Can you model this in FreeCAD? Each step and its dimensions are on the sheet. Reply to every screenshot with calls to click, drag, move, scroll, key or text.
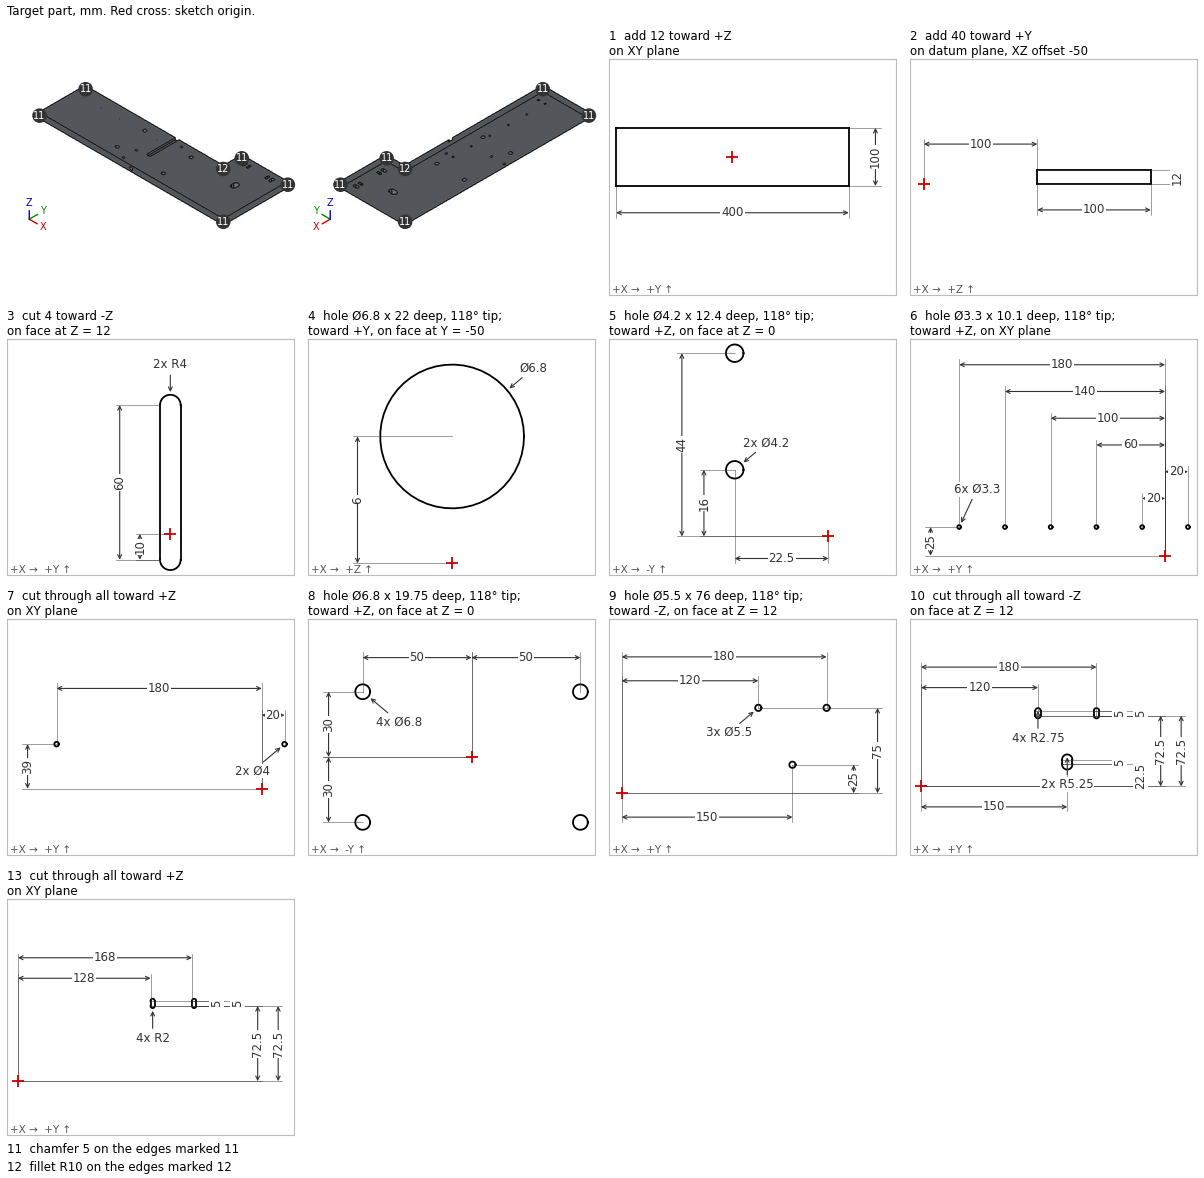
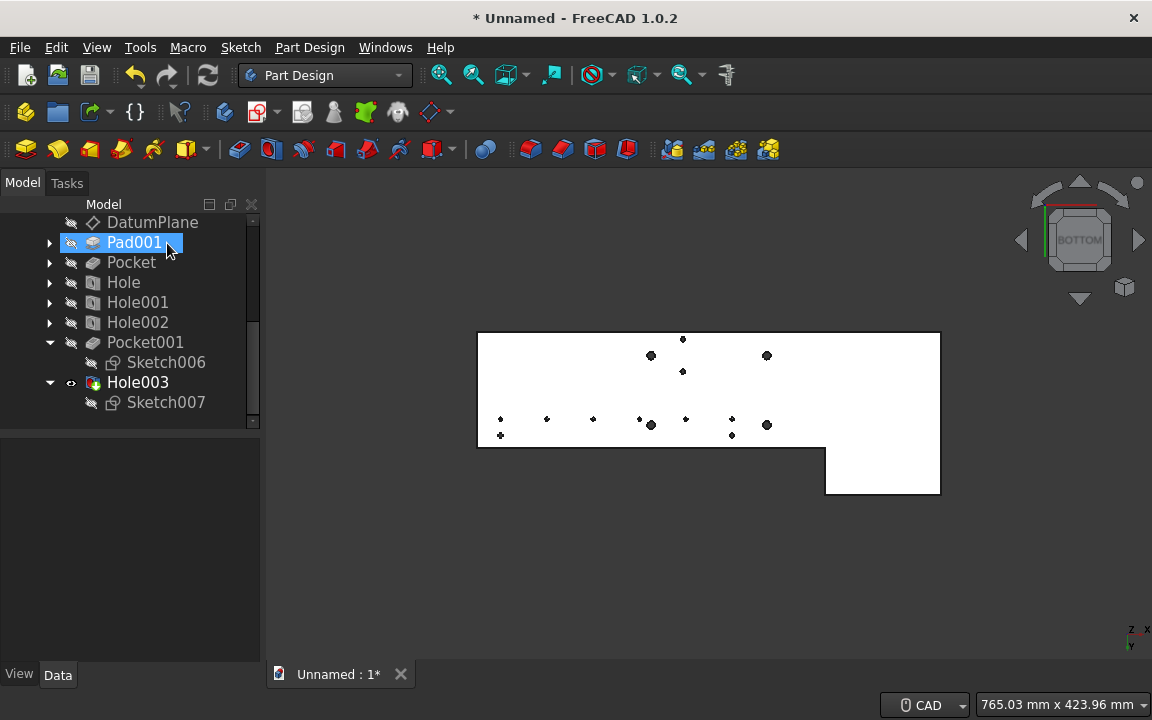
key(0)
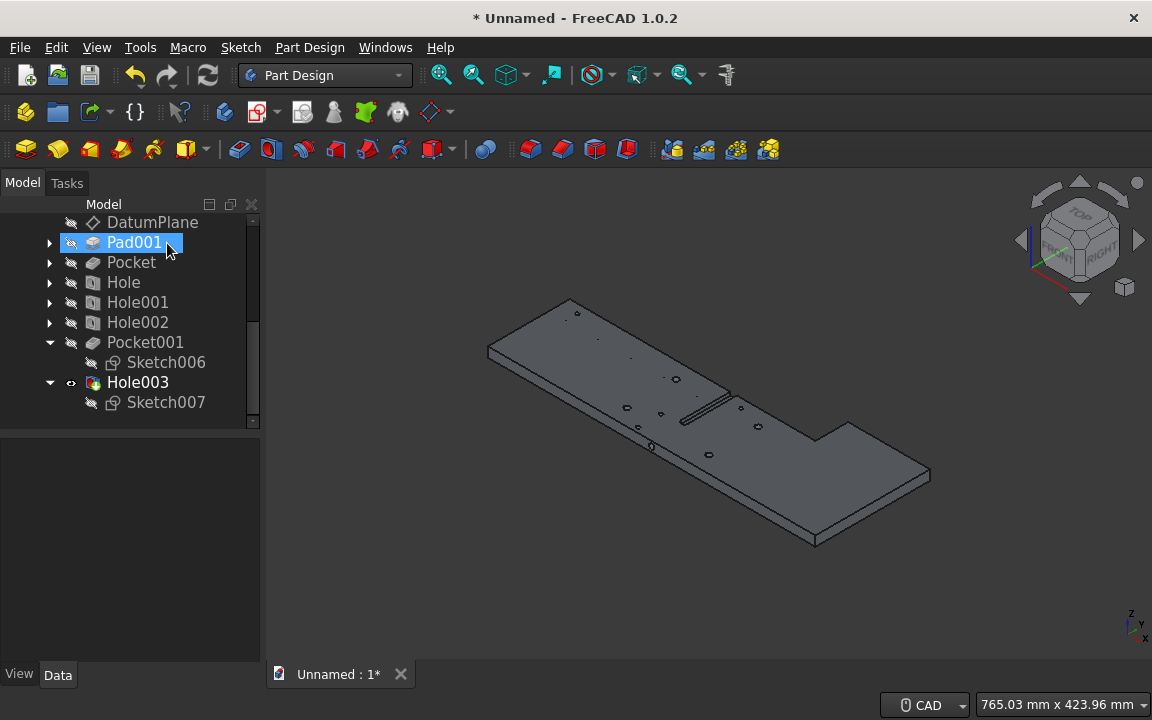
click(786, 470)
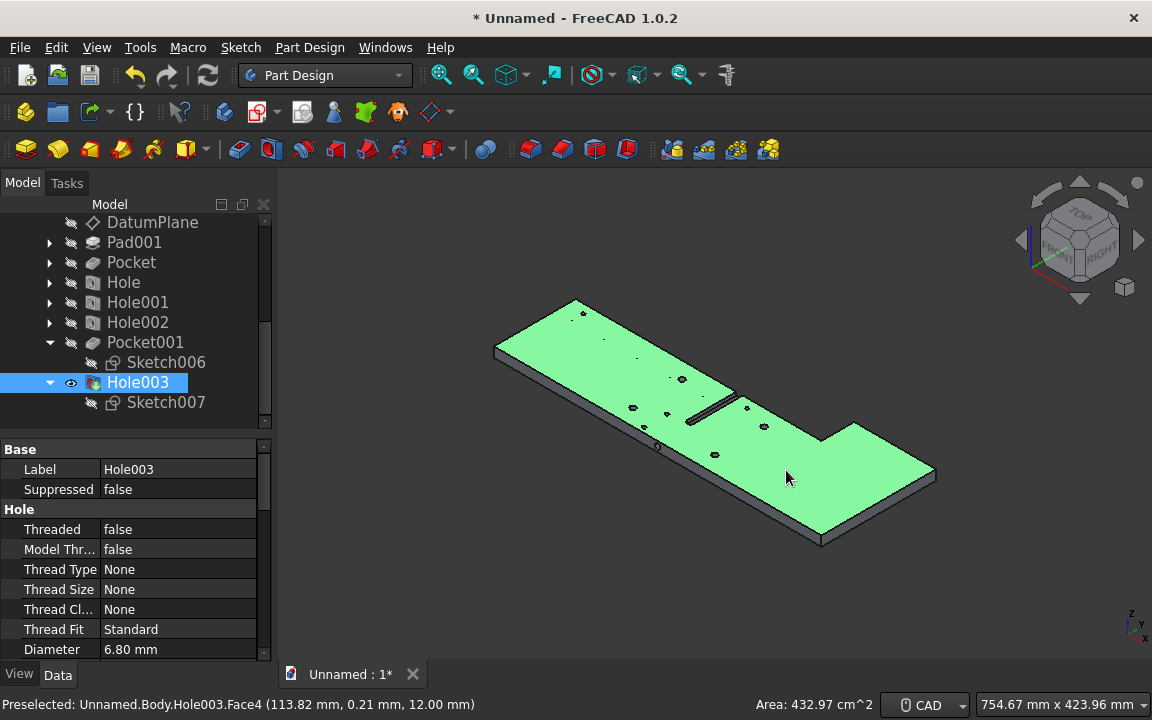
click(258, 112)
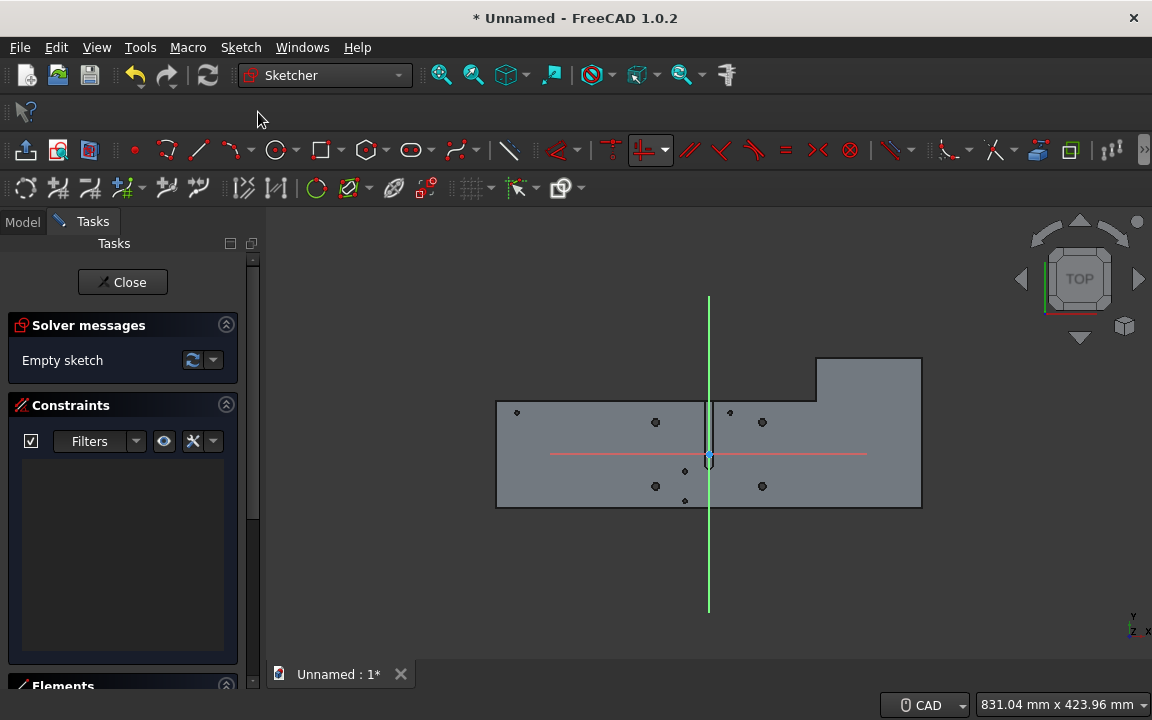
scroll(927, 393, up, 8)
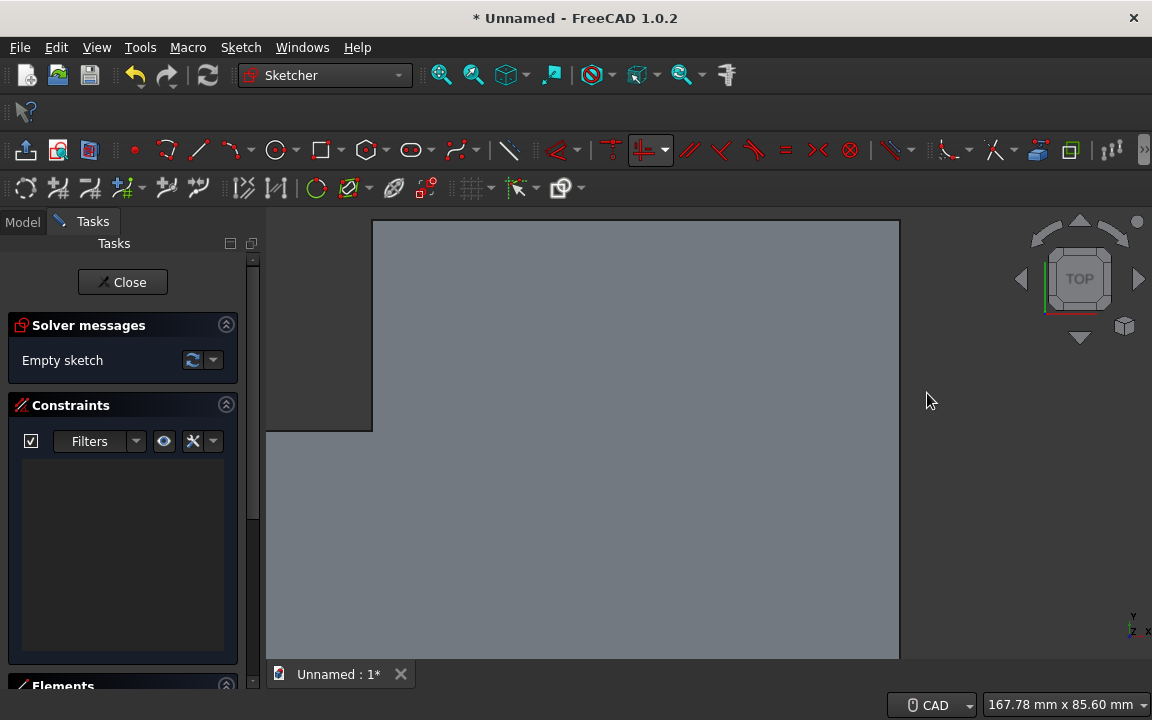
click(276, 150)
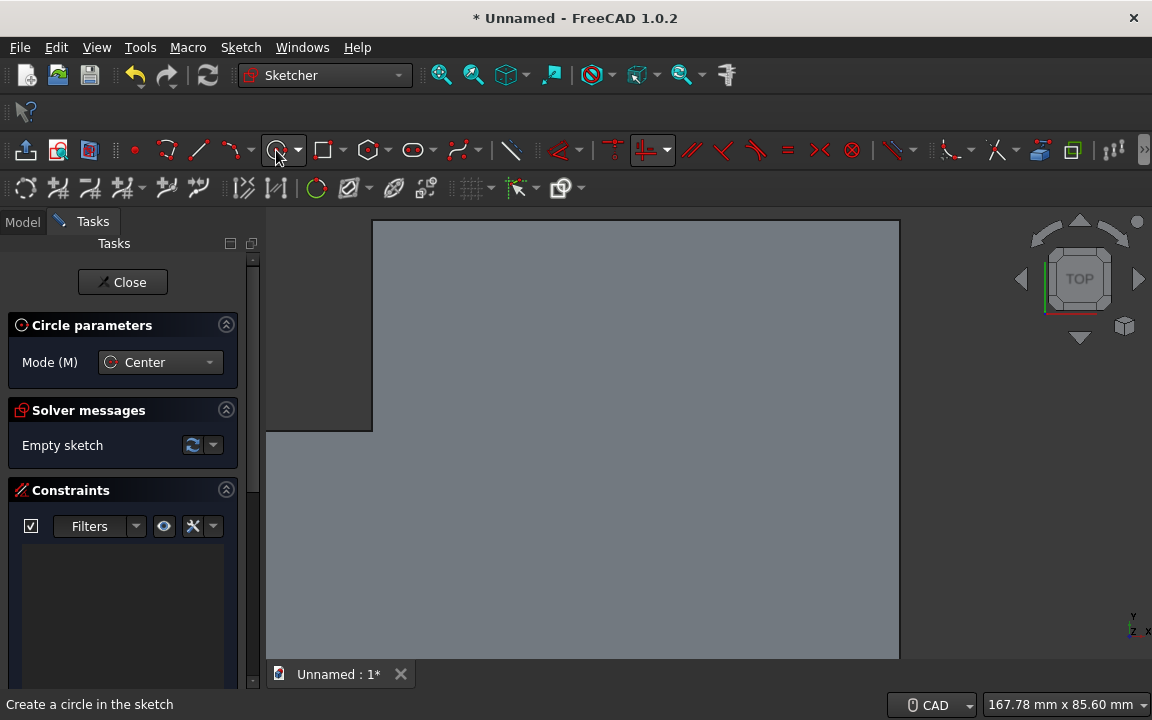
scroll(478, 299, up, 3)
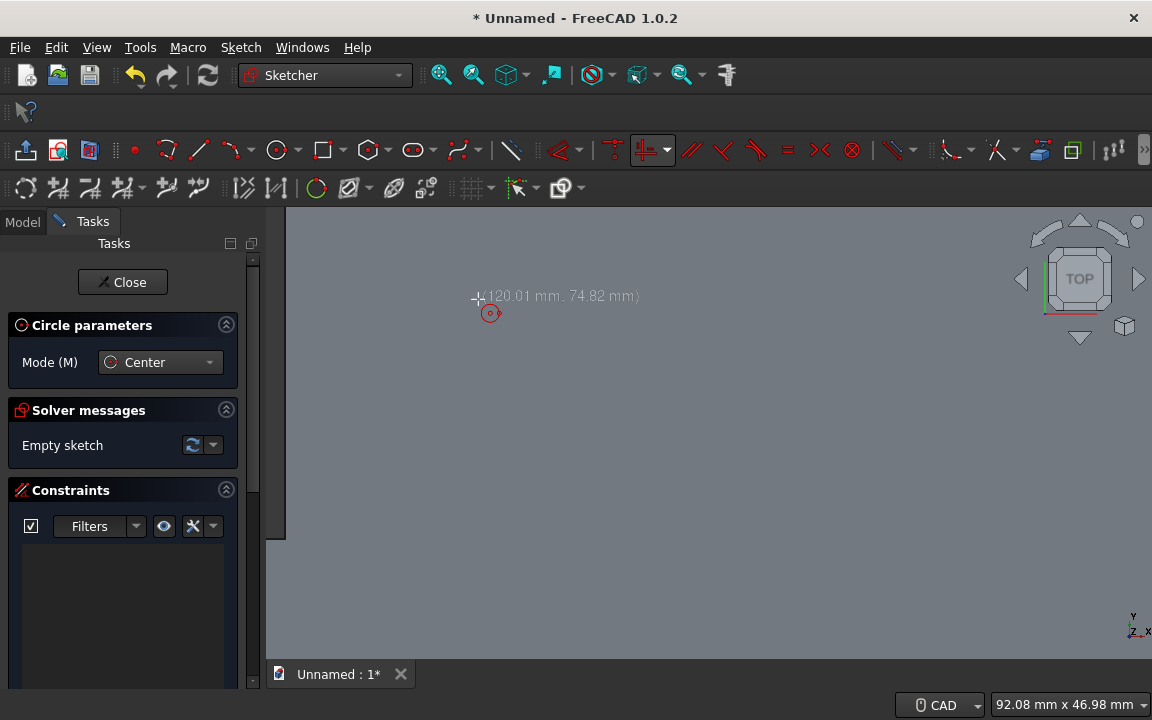
click(478, 299)
move(496, 280)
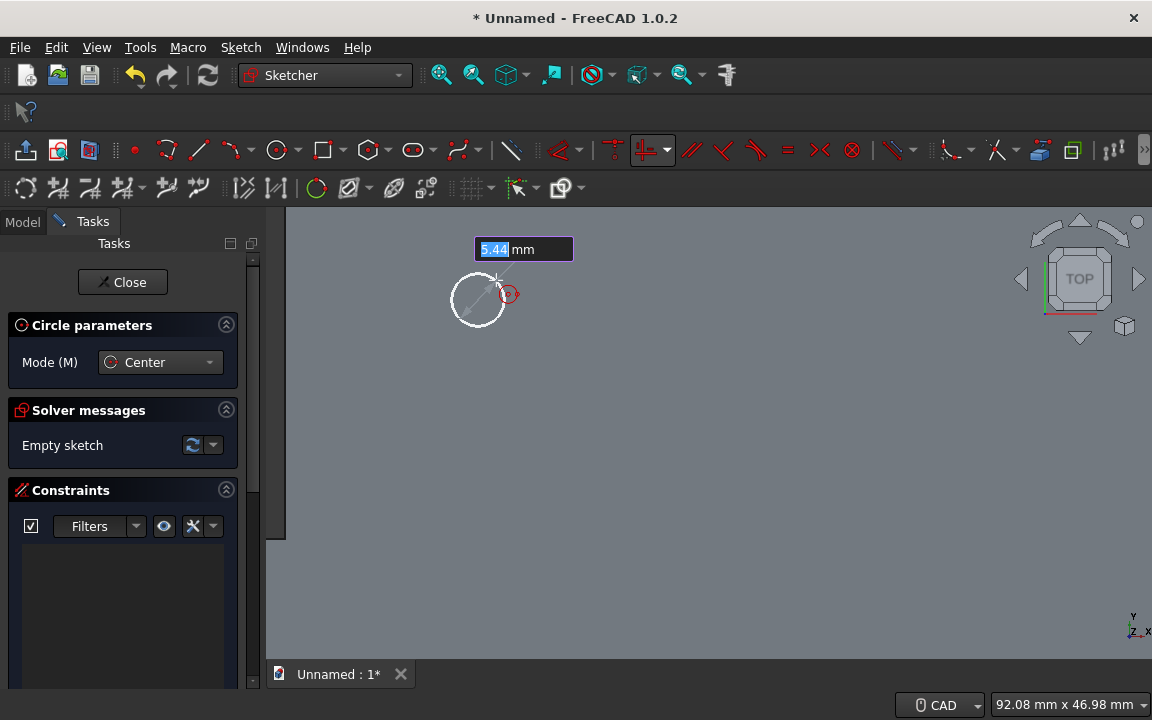
text(5.5)
key(Return)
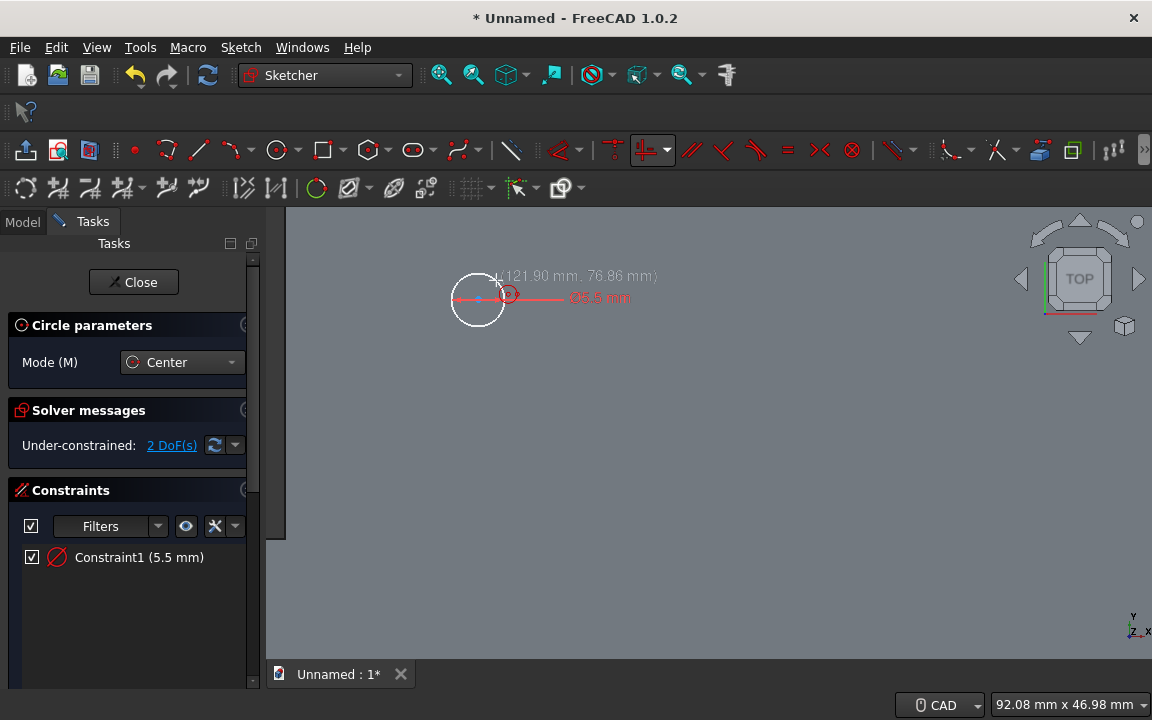
scroll(487, 303, down, 3)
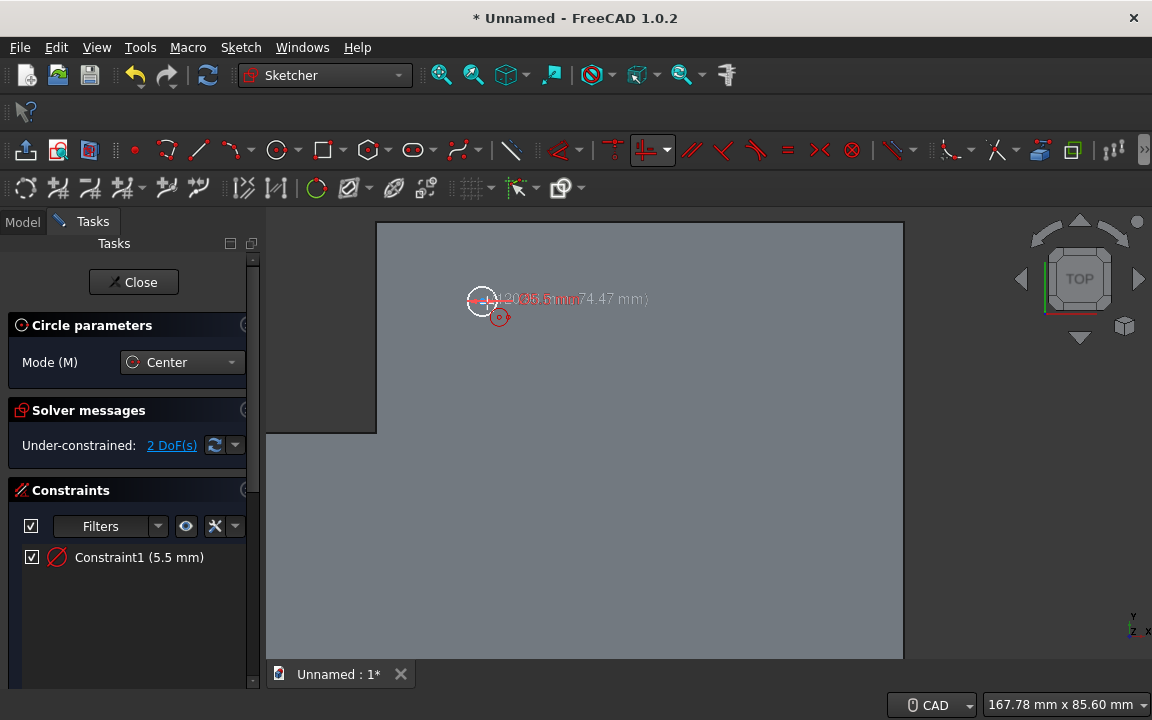
scroll(799, 301, up, 3)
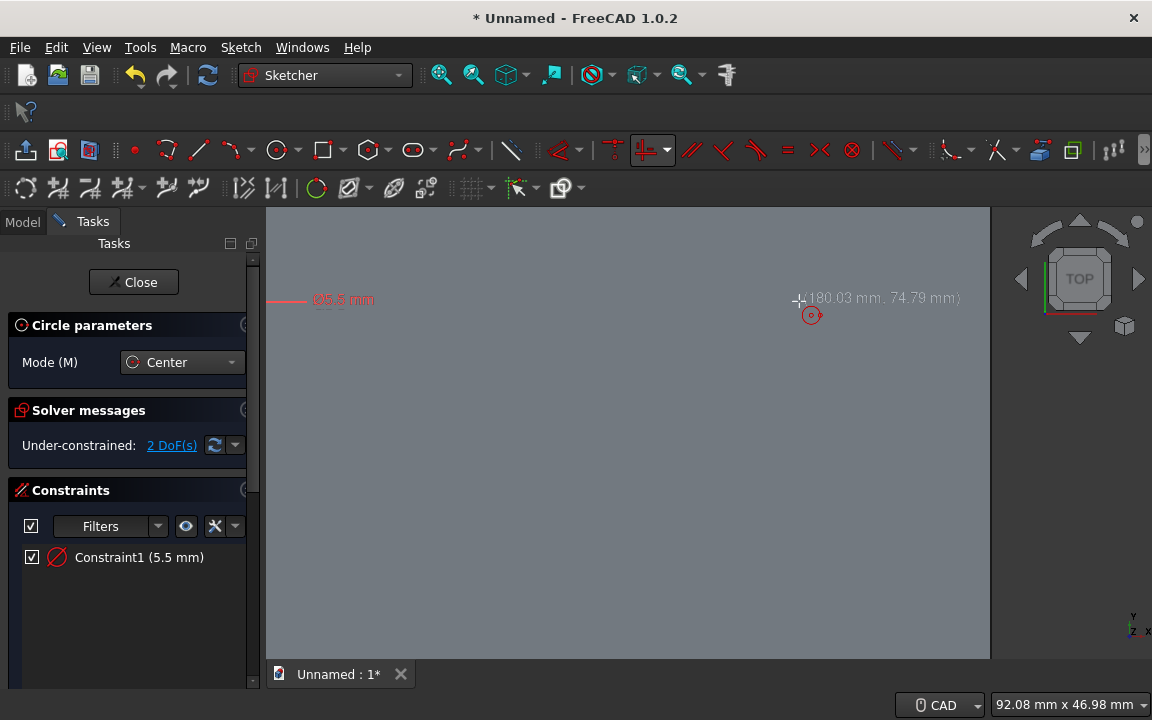
click(798, 301)
move(817, 282)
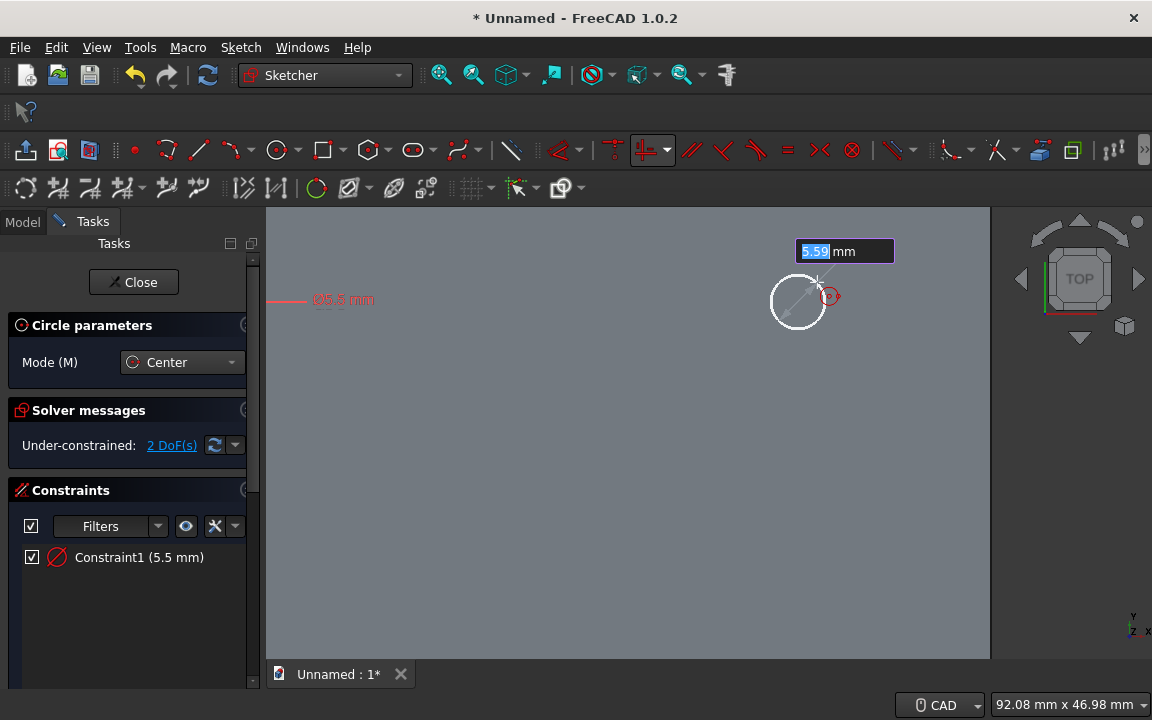
text(5.5)
key(Return)